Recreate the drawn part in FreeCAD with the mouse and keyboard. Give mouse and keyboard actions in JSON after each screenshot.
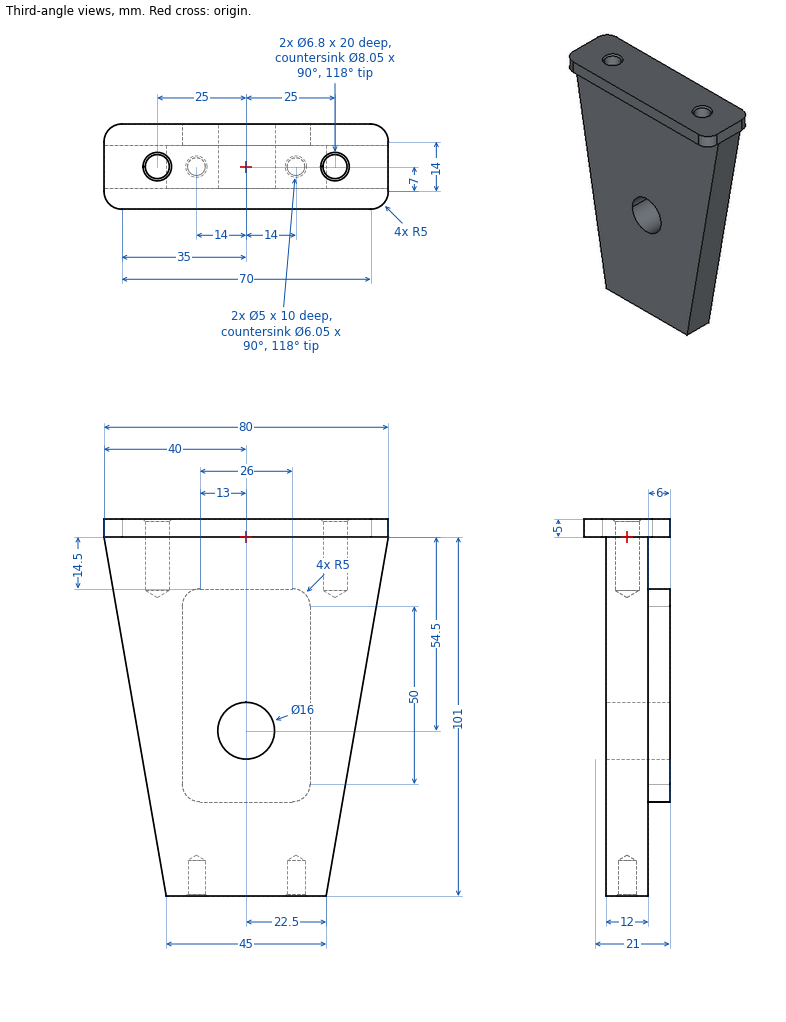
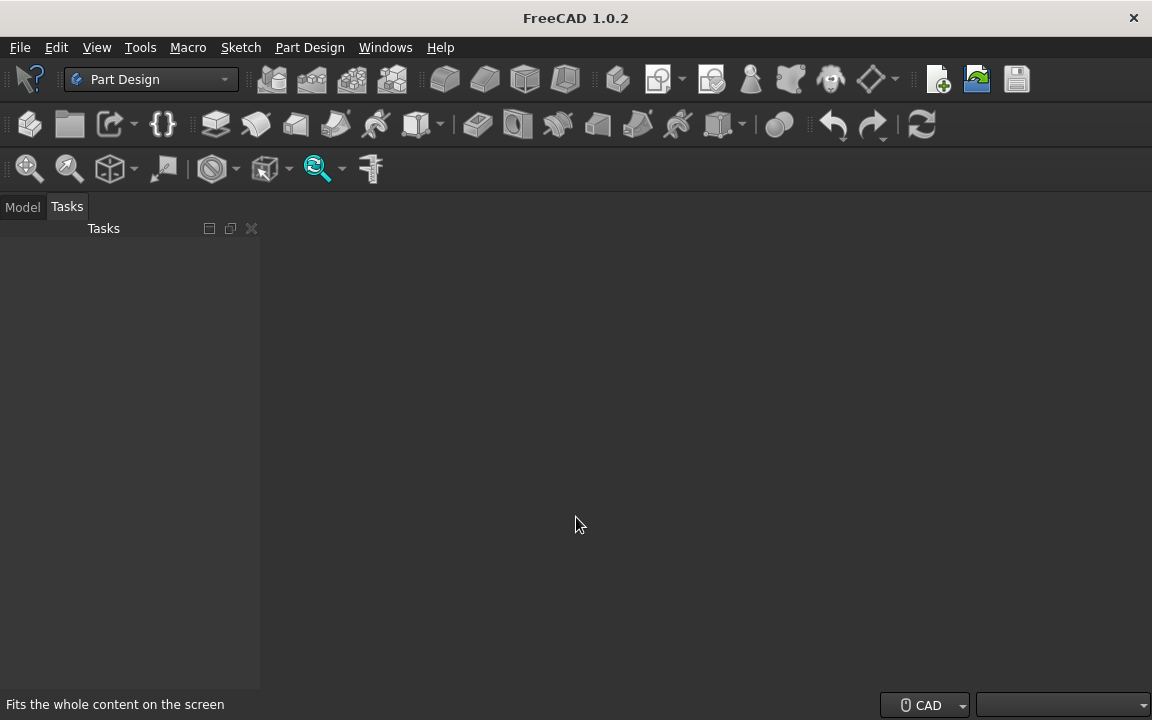
{"action": "key", "text": "ctrl+n"}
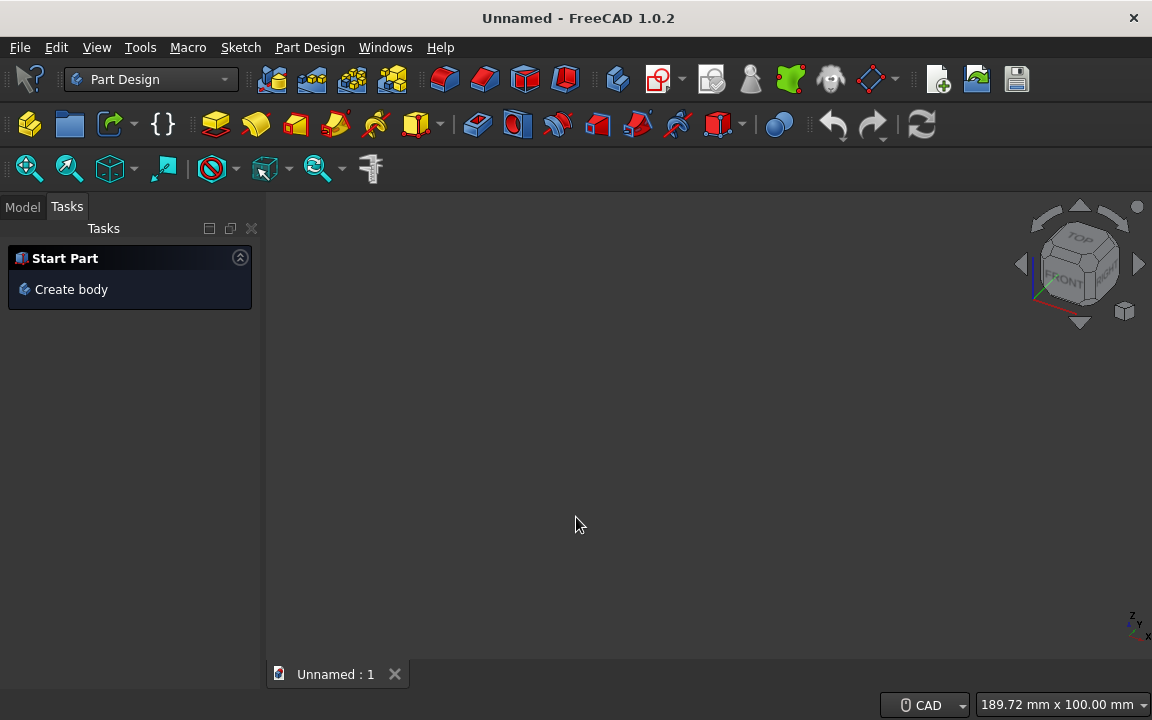
{"action": "left_click", "coordinate": [658, 80]}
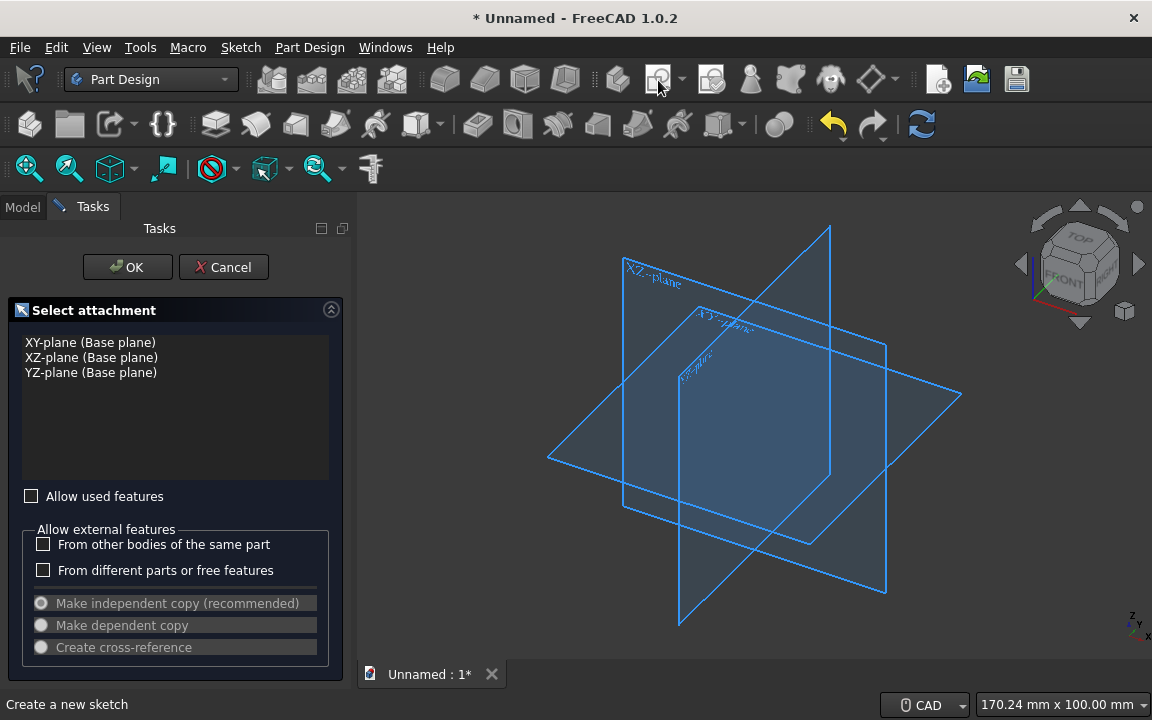
{"action": "left_click", "coordinate": [82, 342]}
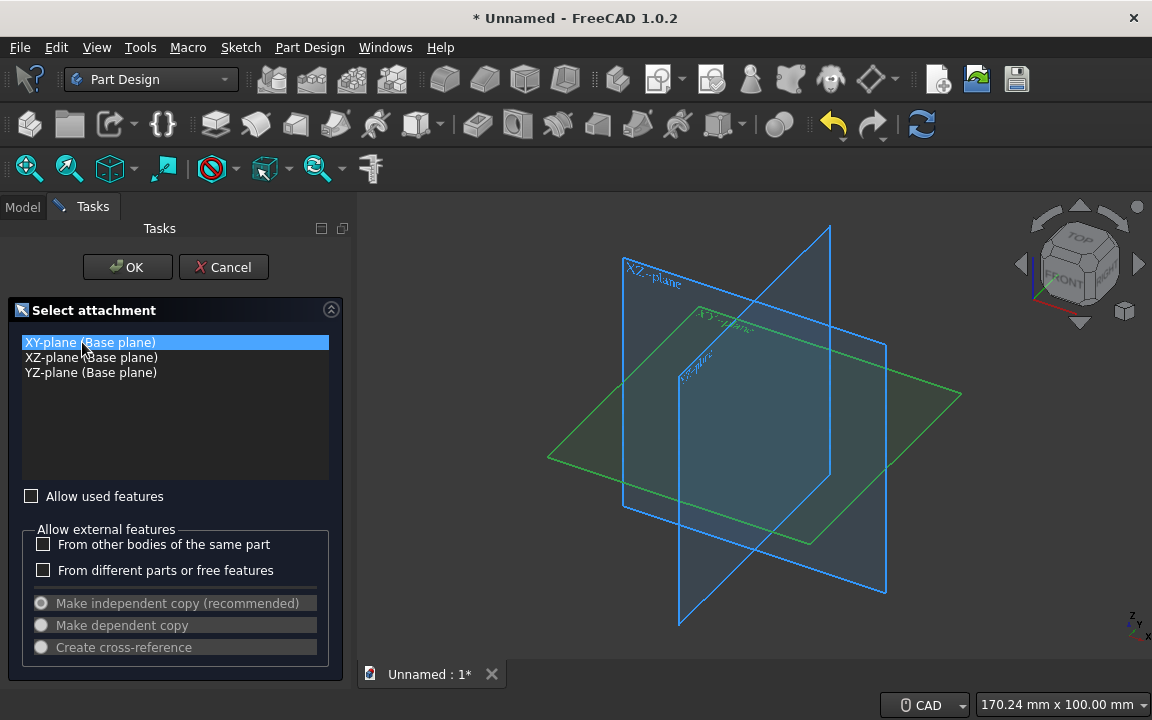
{"action": "left_click", "coordinate": [128, 267]}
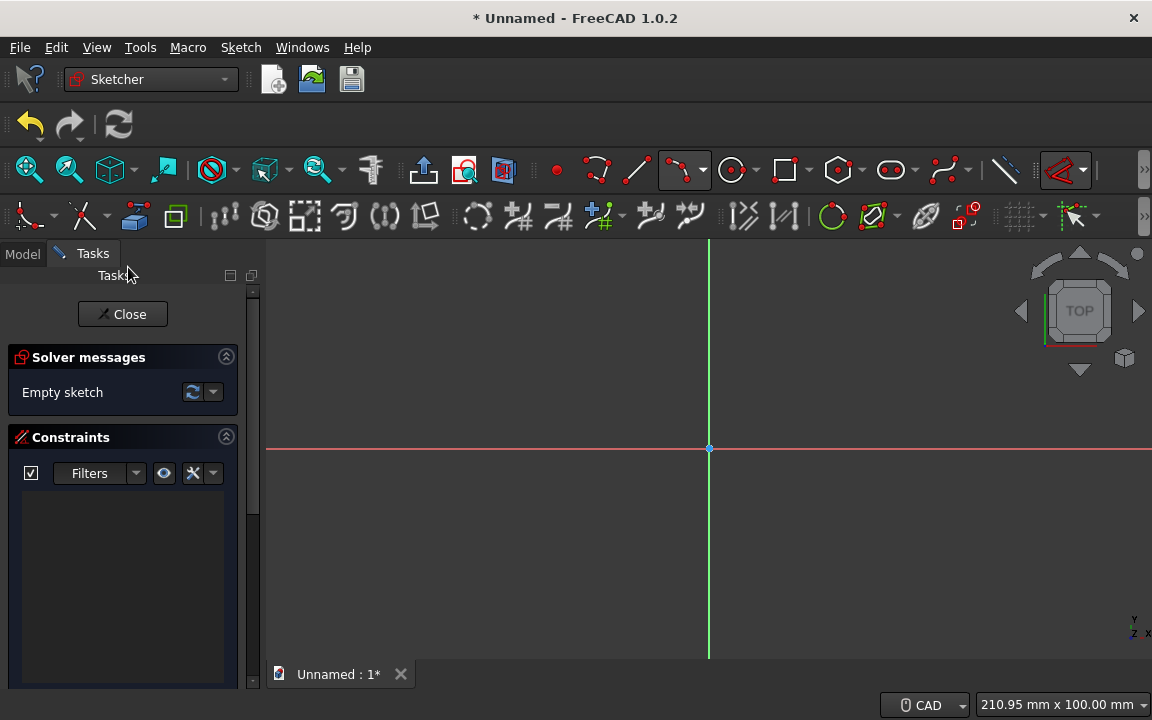
{"action": "scroll", "coordinate": [848, 449], "scroll_direction": "up", "scroll_amount": 2}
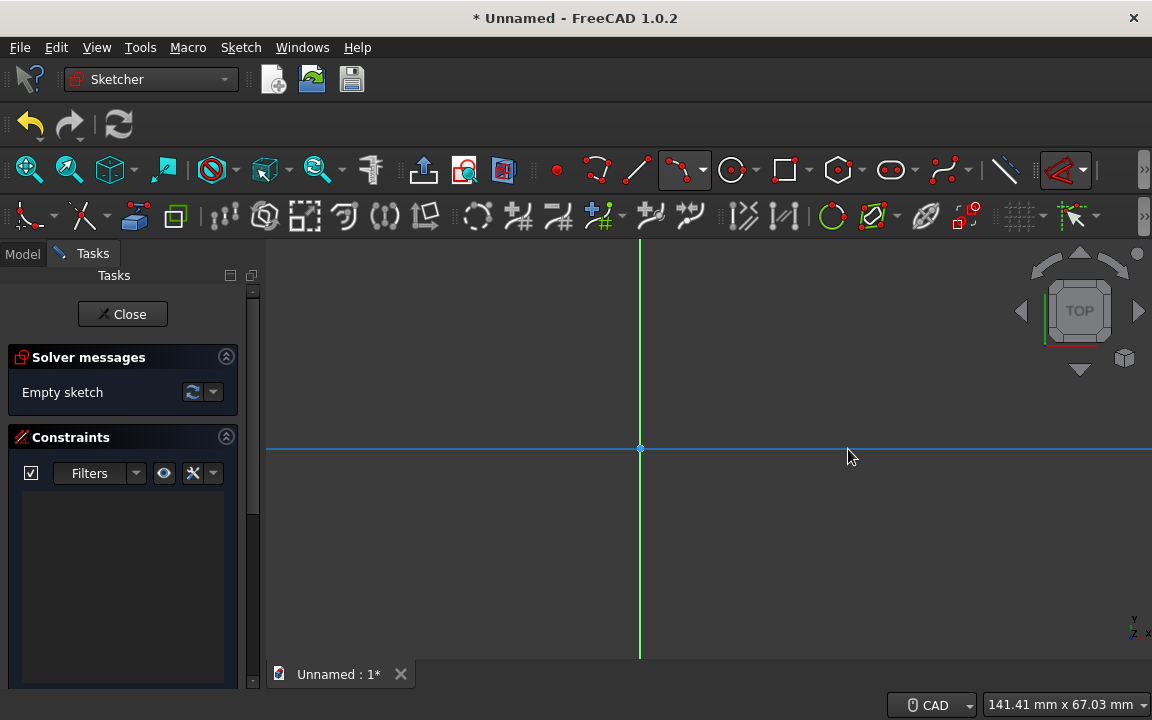
{"action": "key", "text": "g l"}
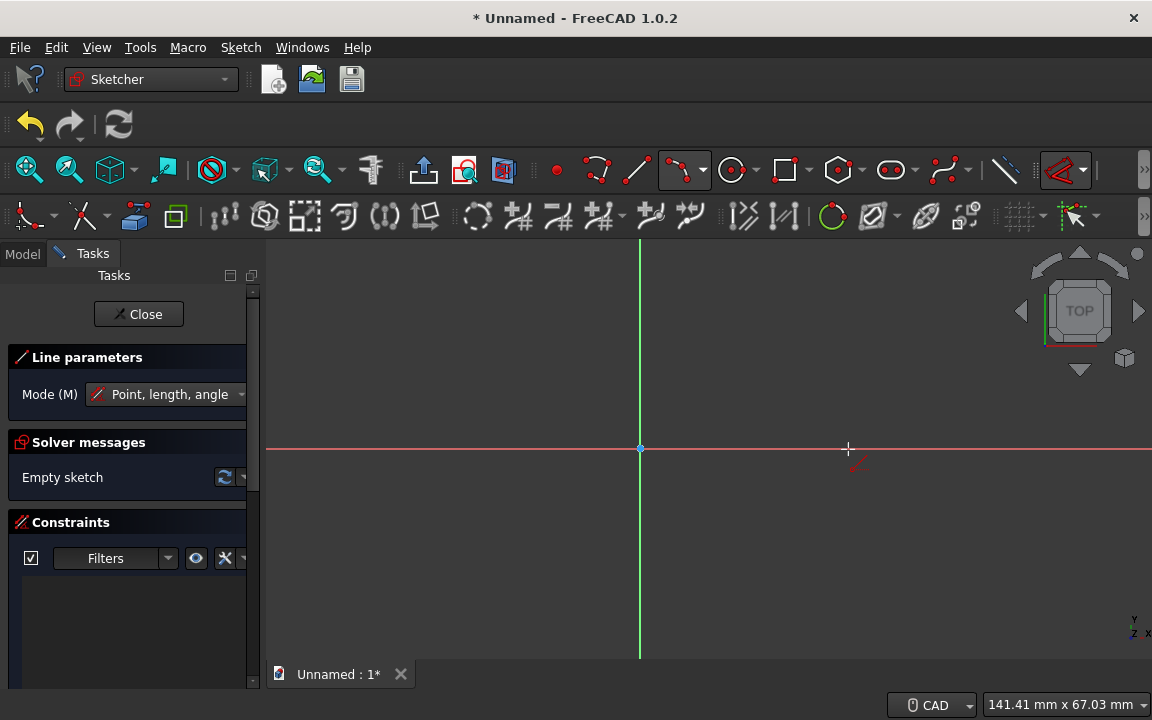
{"action": "left_click", "coordinate": [421, 524]}
{"action": "left_click", "coordinate": [860, 524]}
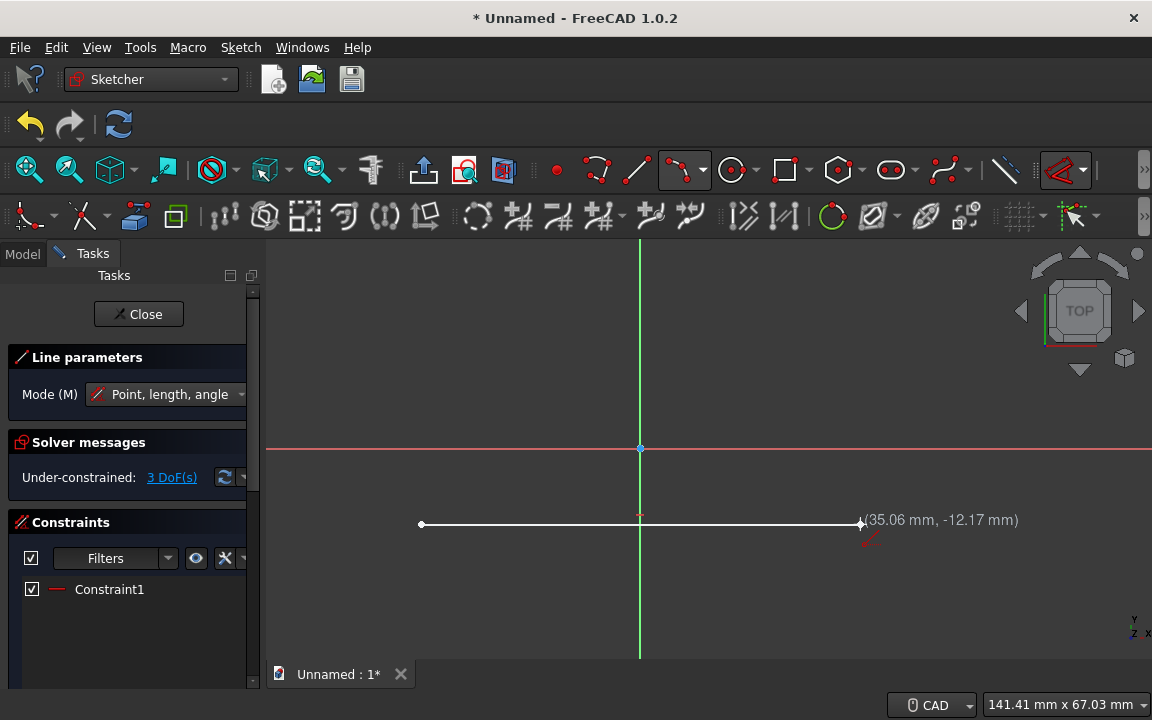
{"action": "left_click", "coordinate": [891, 493]}
{"action": "left_click", "coordinate": [891, 405]}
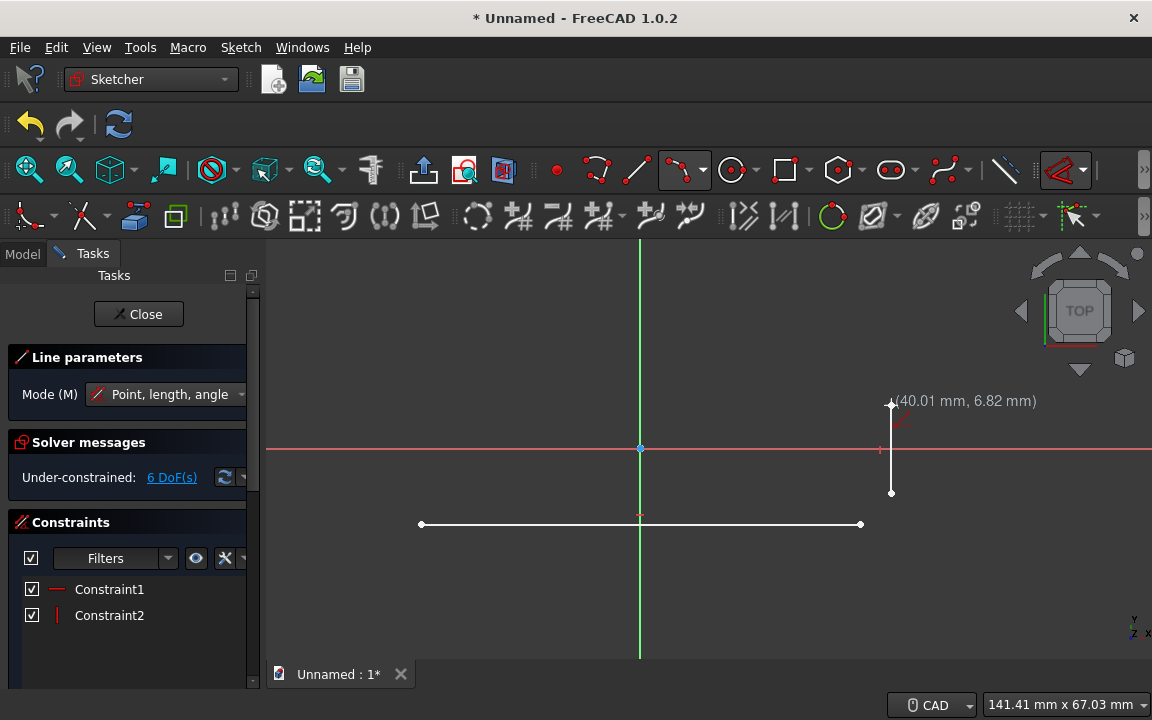
{"action": "left_click", "coordinate": [860, 374]}
{"action": "left_click", "coordinate": [421, 374]}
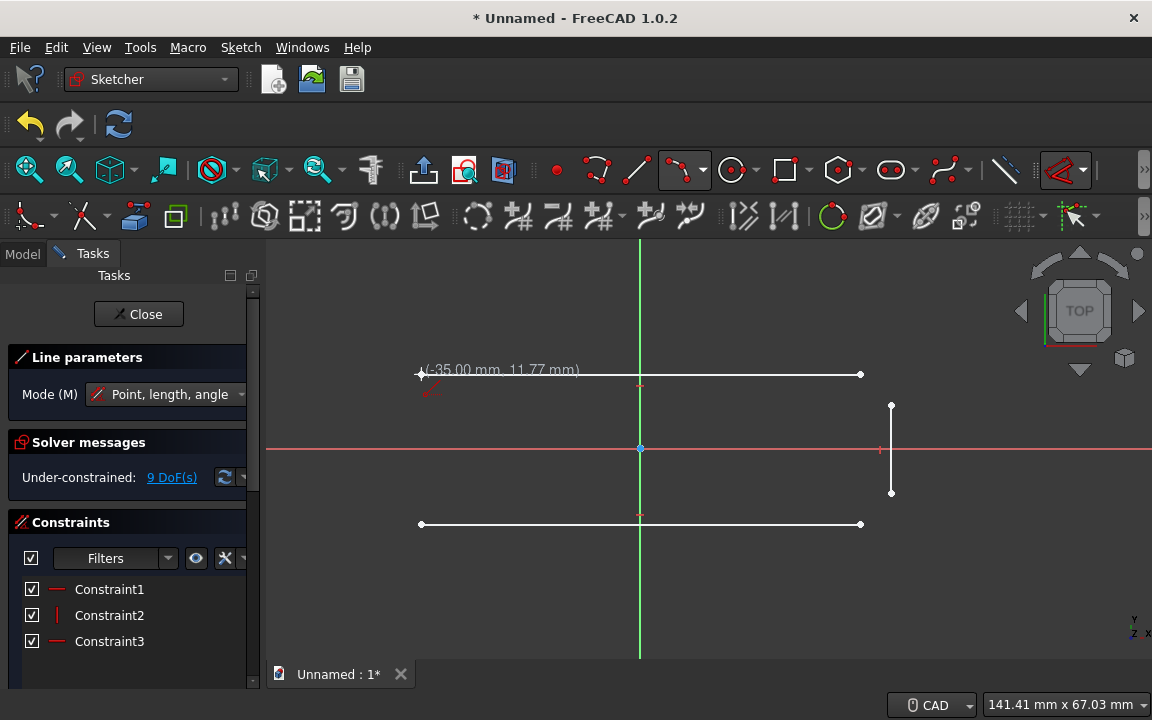
{"action": "left_click", "coordinate": [390, 405]}
{"action": "left_click", "coordinate": [390, 493]}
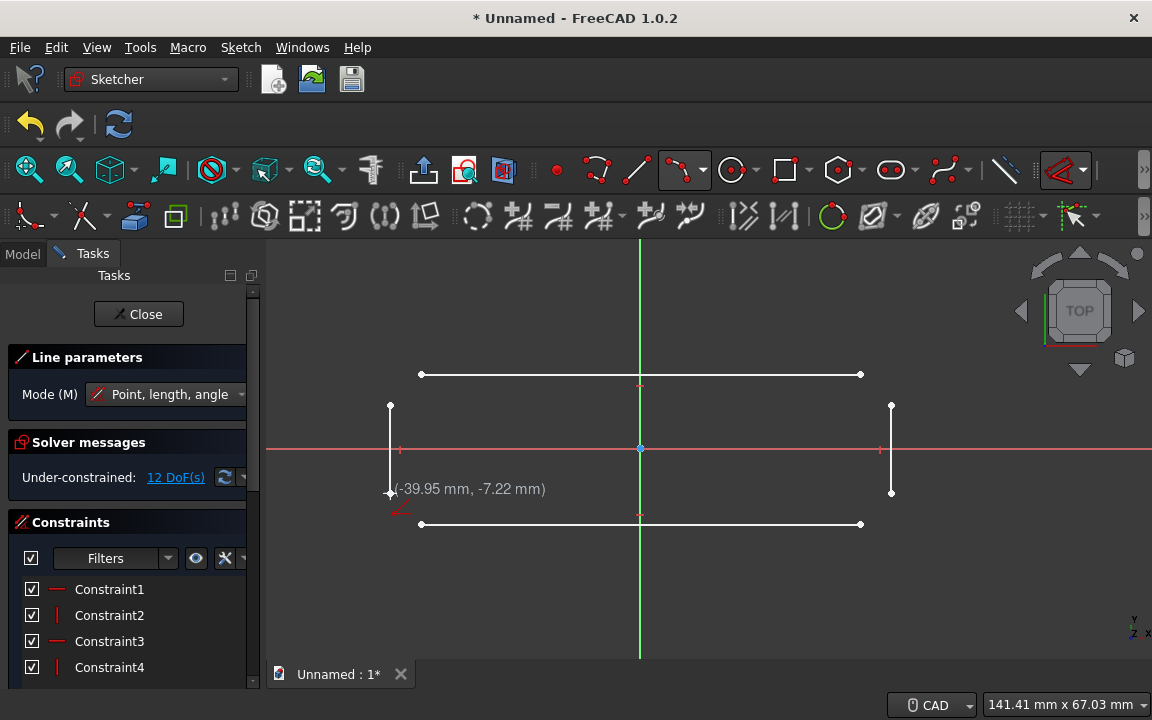
{"action": "left_click", "coordinate": [678, 170]}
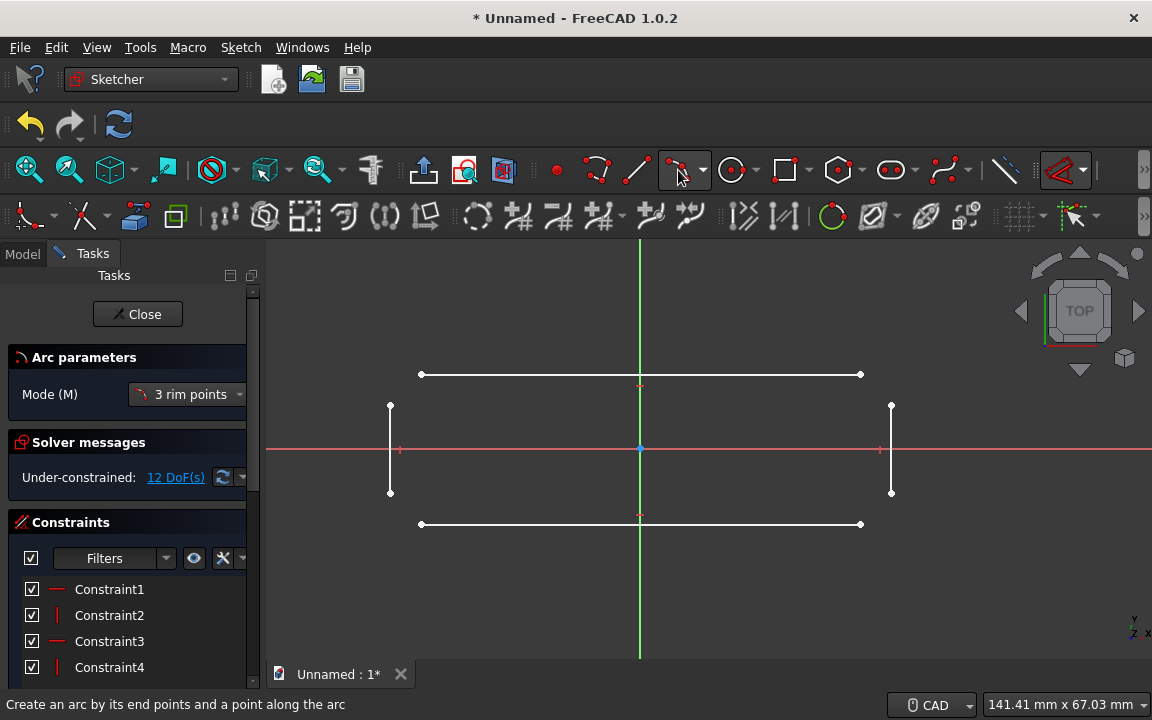
{"action": "left_click", "coordinate": [860, 525]}
{"action": "left_click", "coordinate": [891, 494]}